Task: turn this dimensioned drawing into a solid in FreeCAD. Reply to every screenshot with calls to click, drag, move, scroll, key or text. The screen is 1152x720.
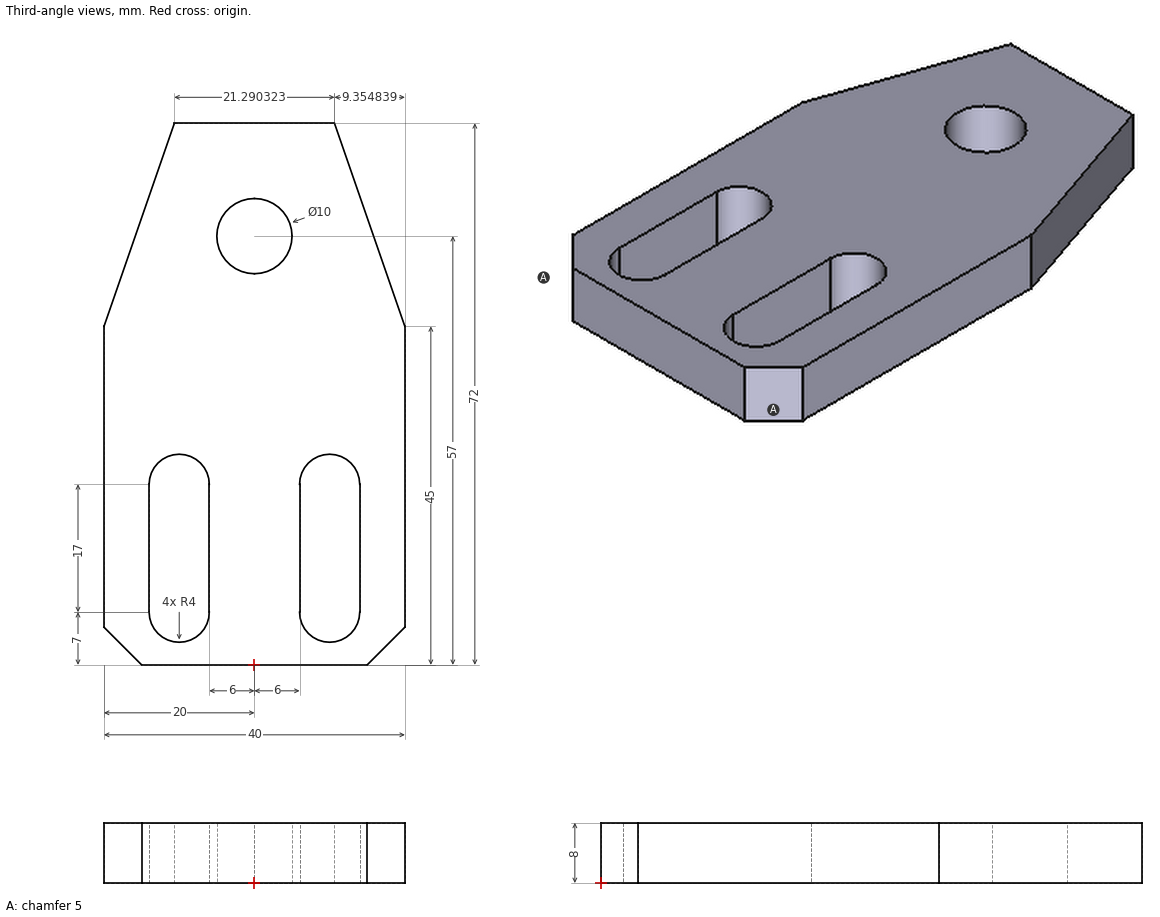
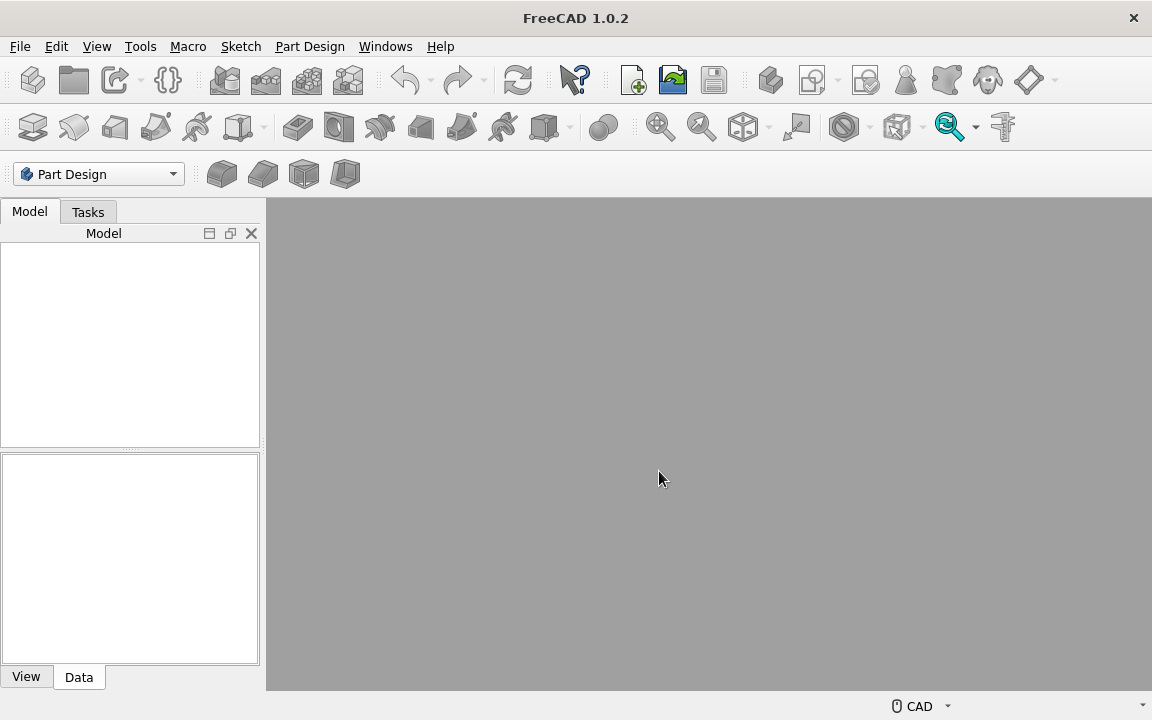
click(632, 80)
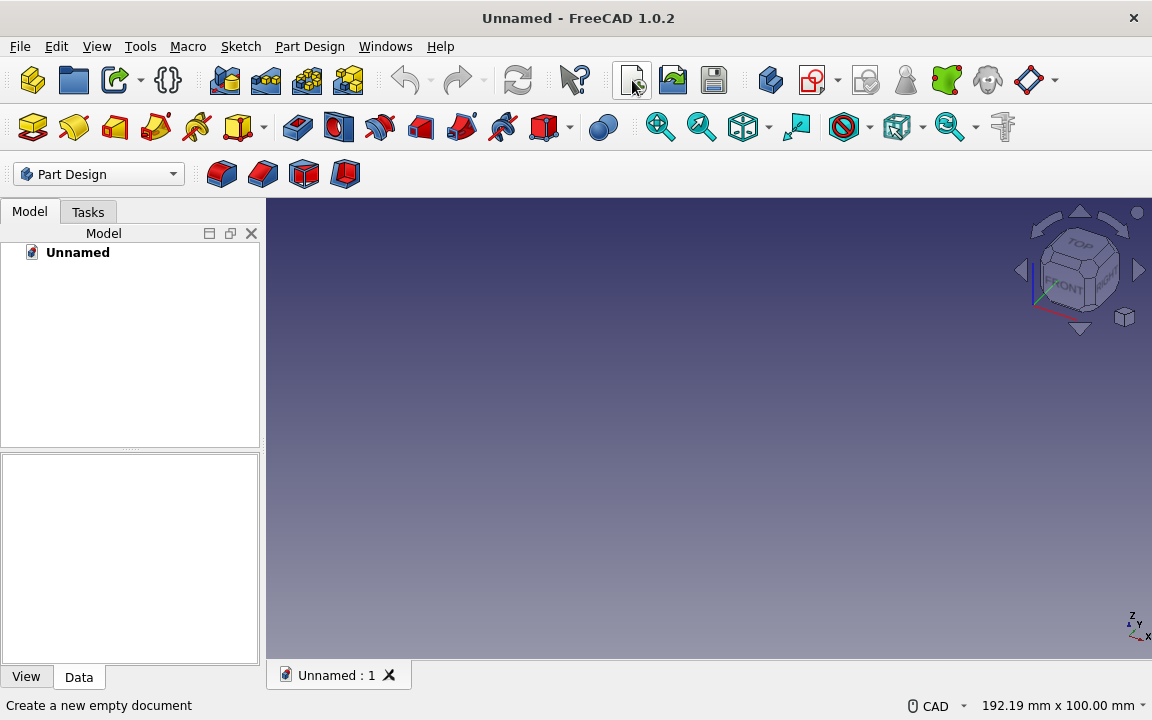
click(812, 80)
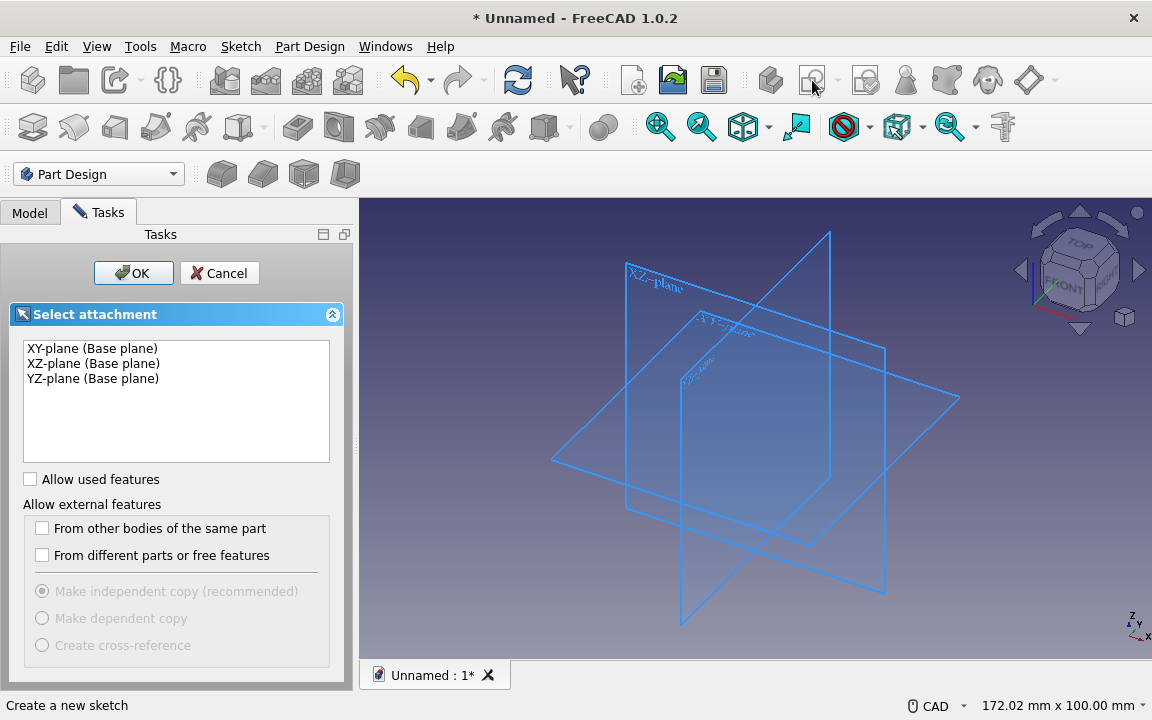
click(84, 348)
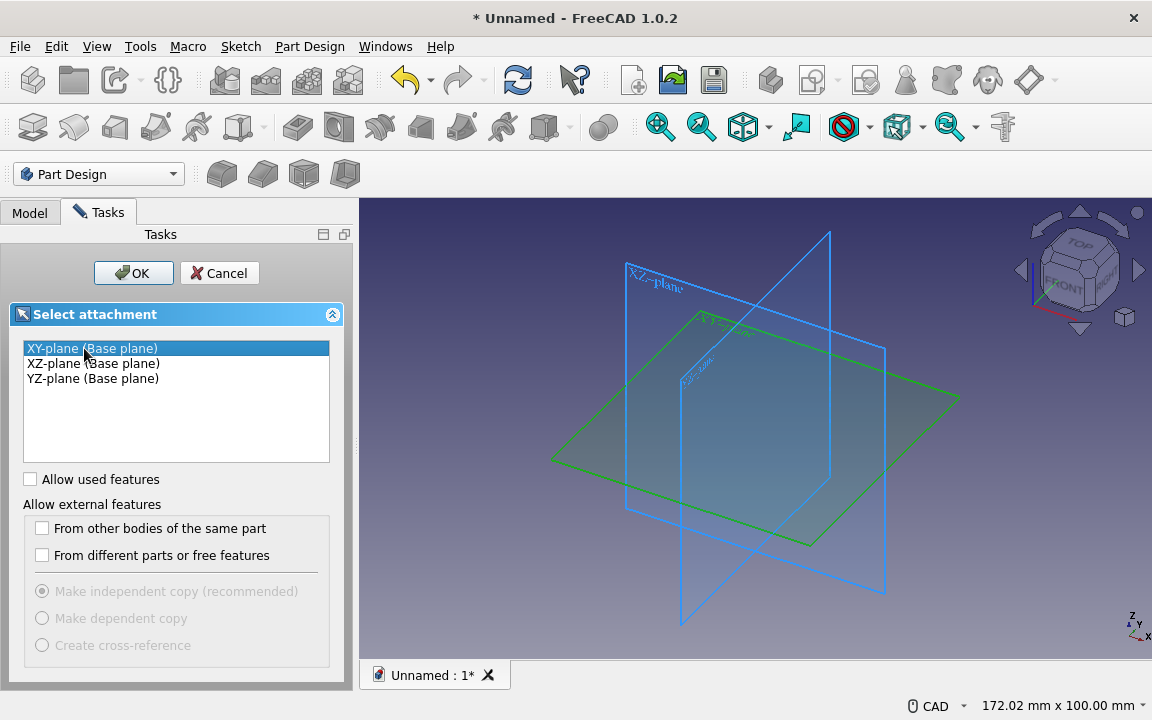
click(134, 273)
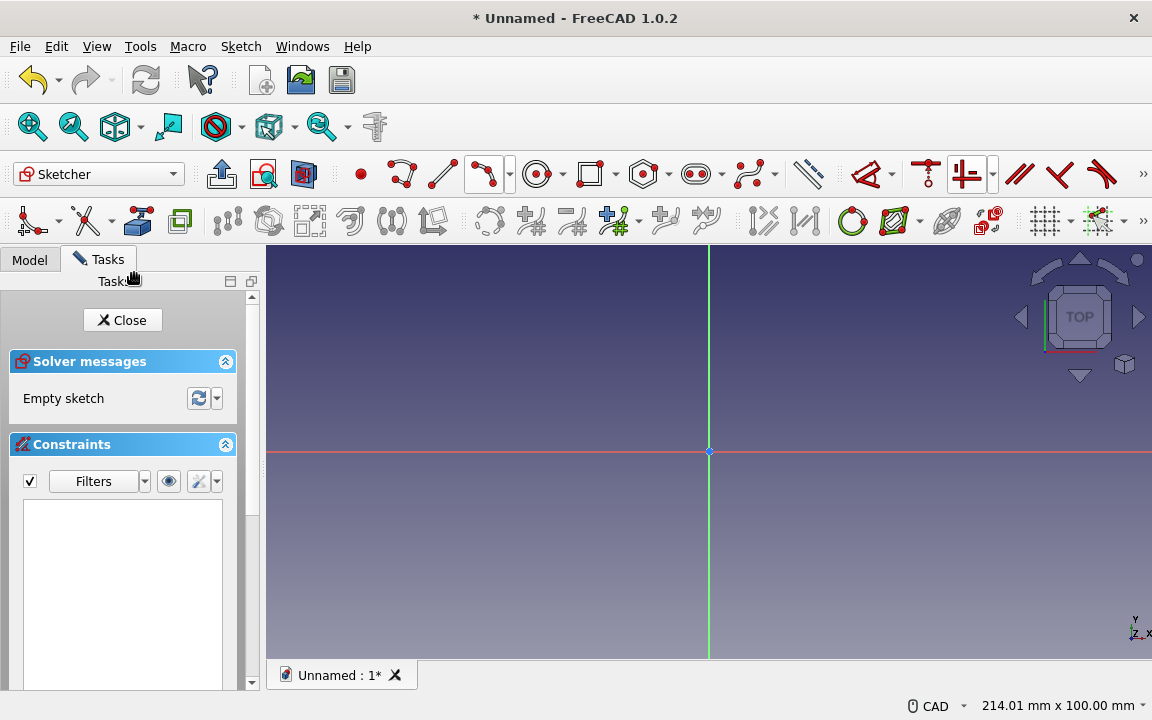
scroll(501, 631, down, 2)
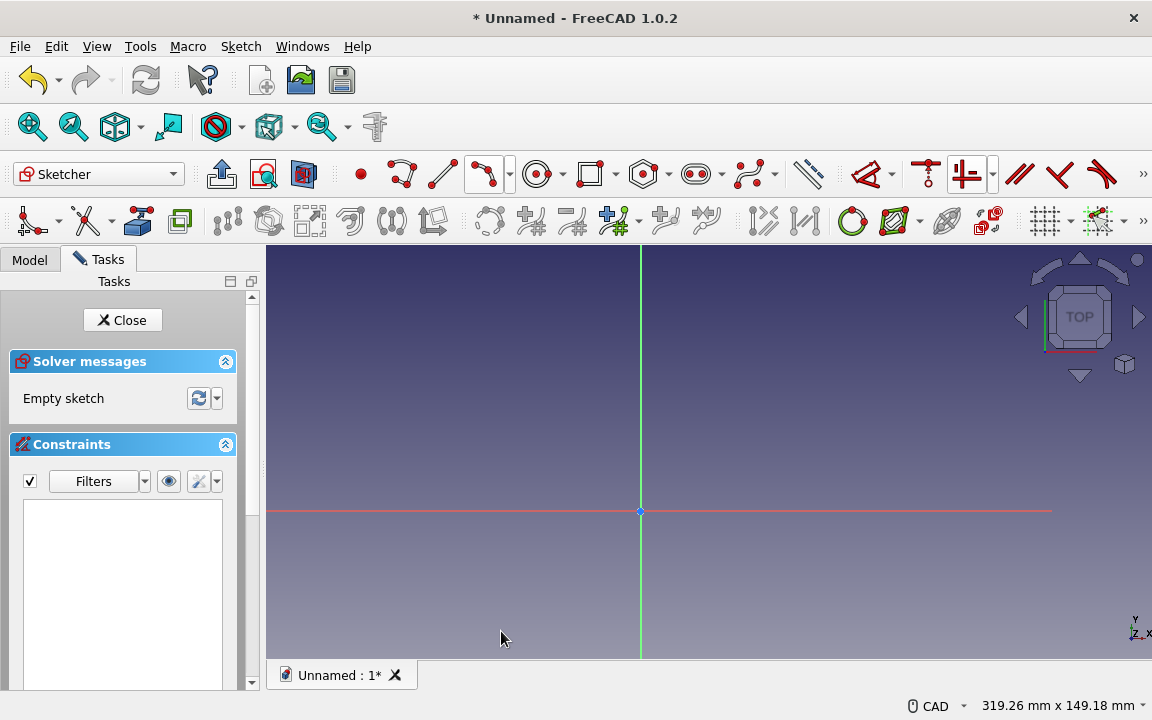
click(402, 174)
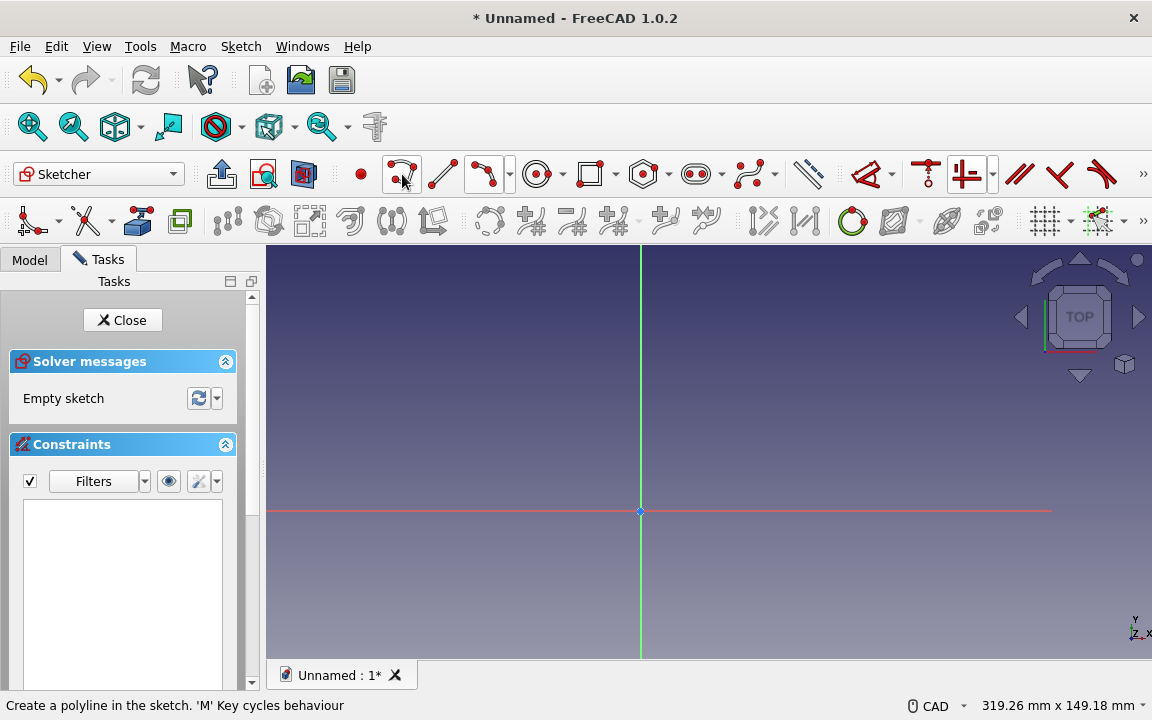
click(585, 511)
click(696, 502)
click(696, 386)
click(670, 312)
click(611, 312)
click(585, 386)
click(585, 511)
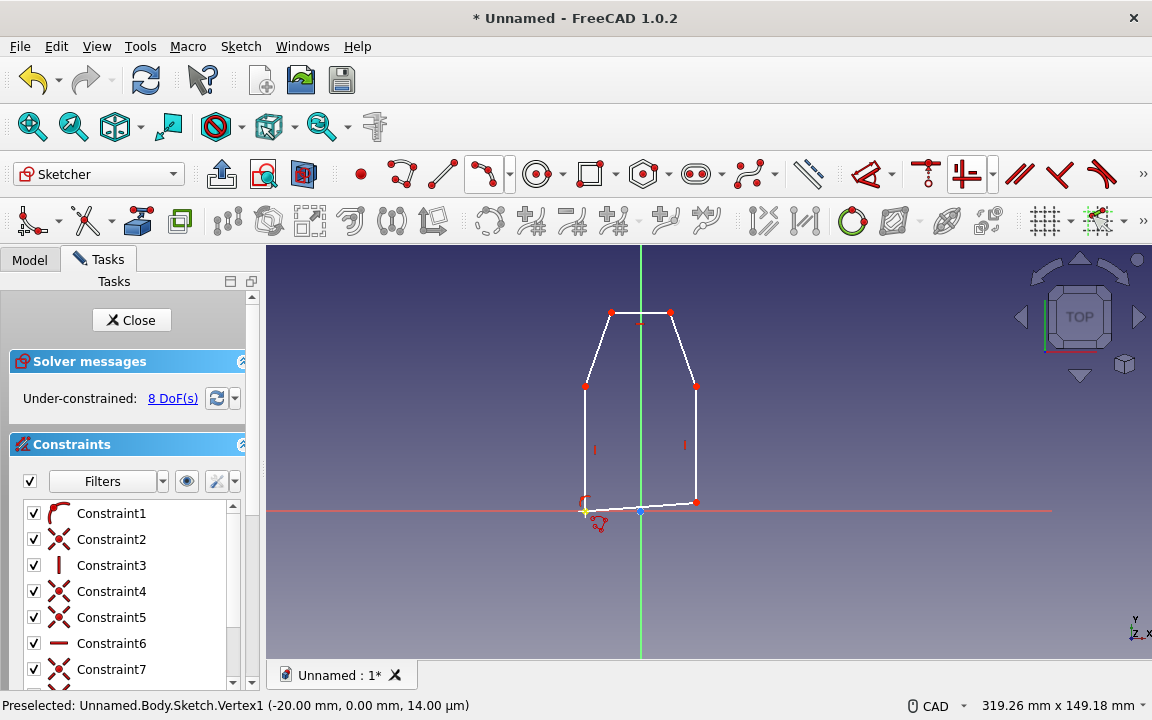
click(696, 174)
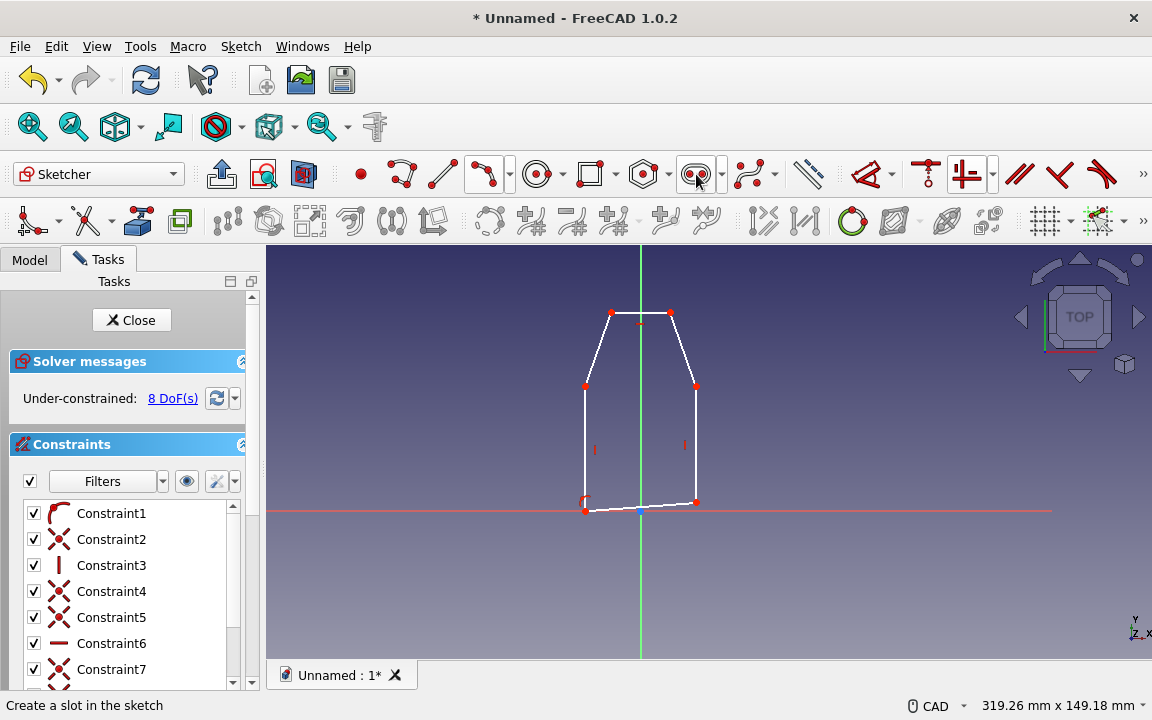
scroll(613, 492, up, 4)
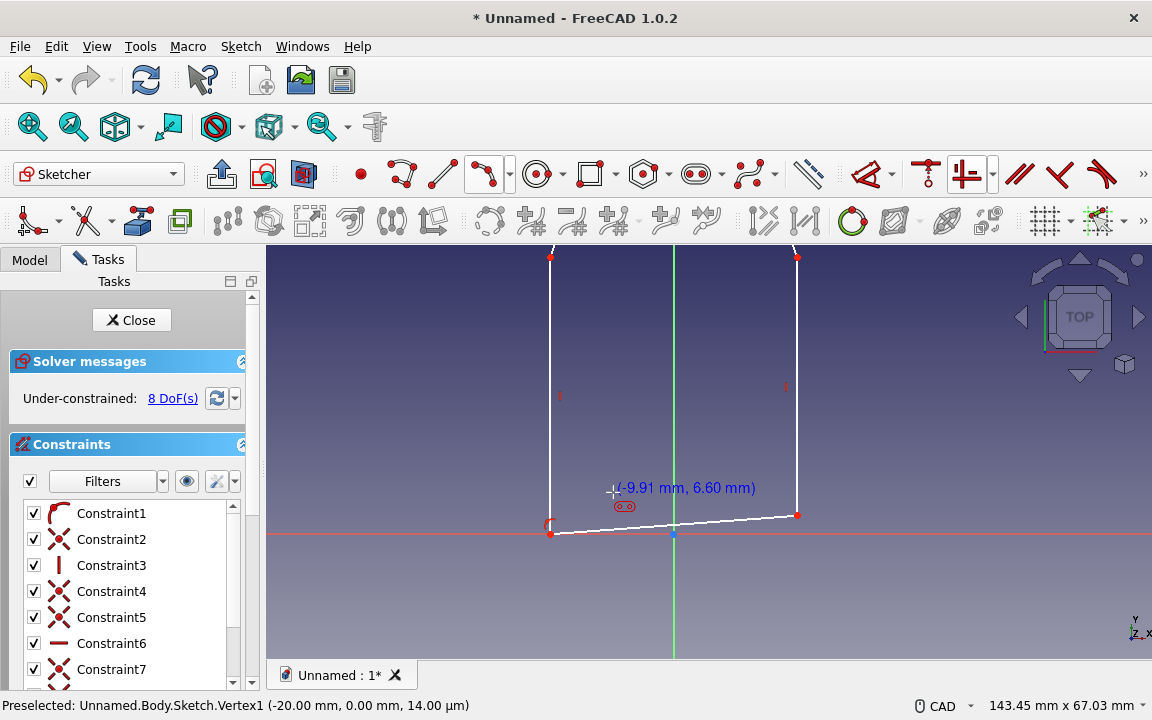
click(612, 491)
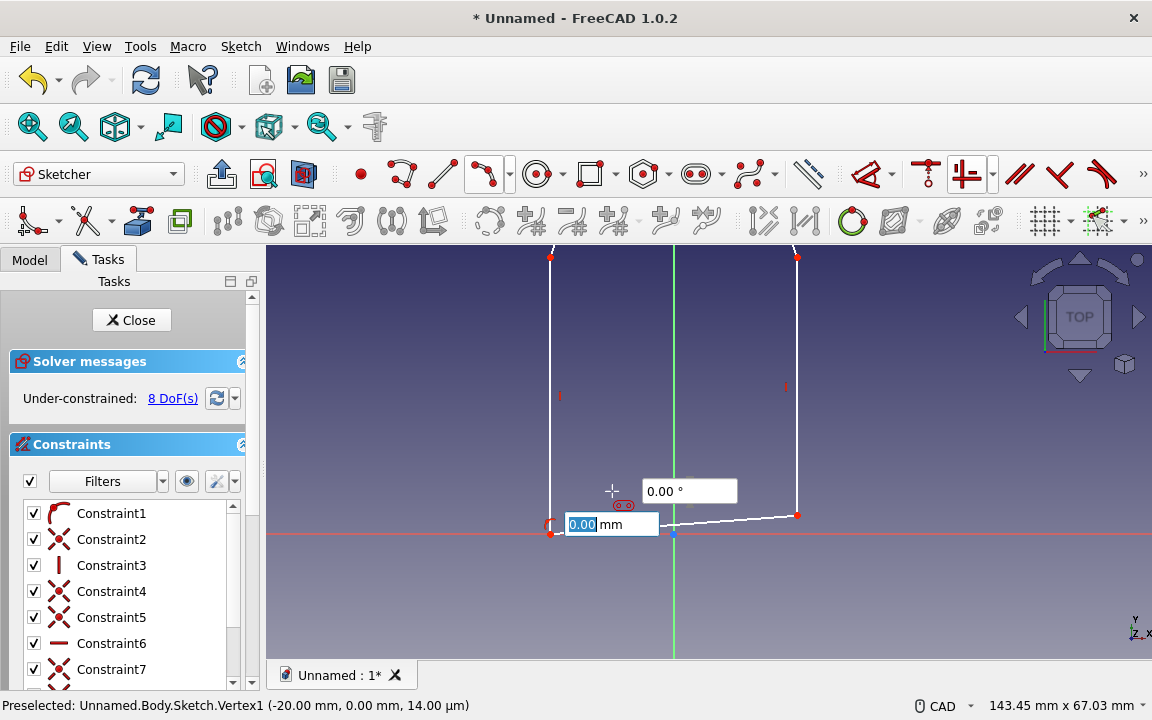
click(612, 386)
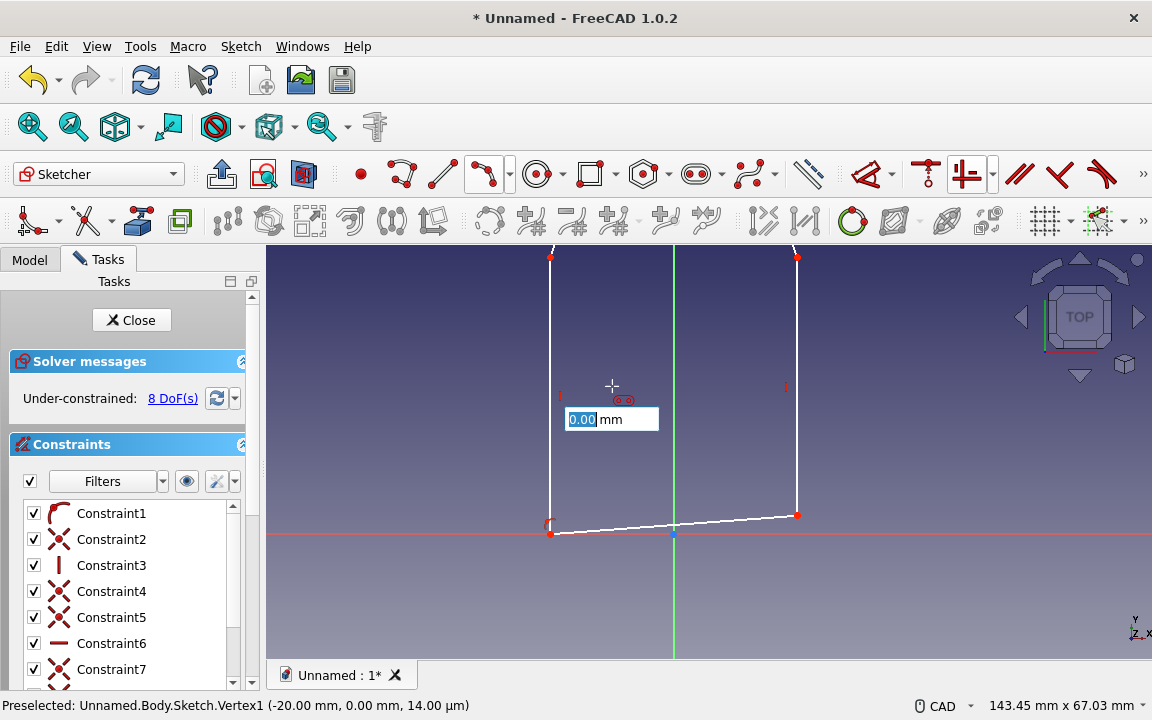
click(637, 439)